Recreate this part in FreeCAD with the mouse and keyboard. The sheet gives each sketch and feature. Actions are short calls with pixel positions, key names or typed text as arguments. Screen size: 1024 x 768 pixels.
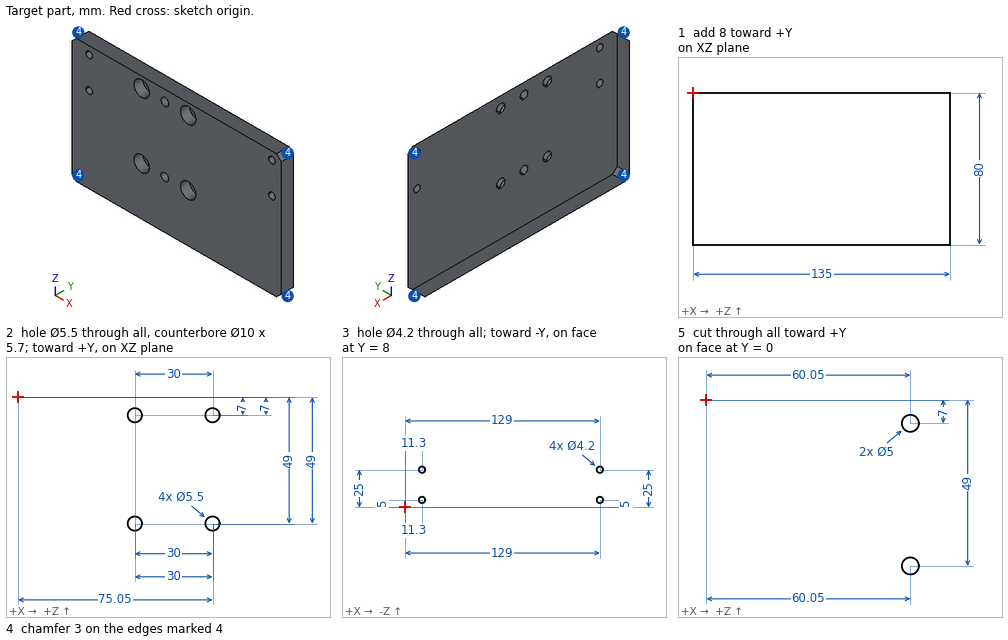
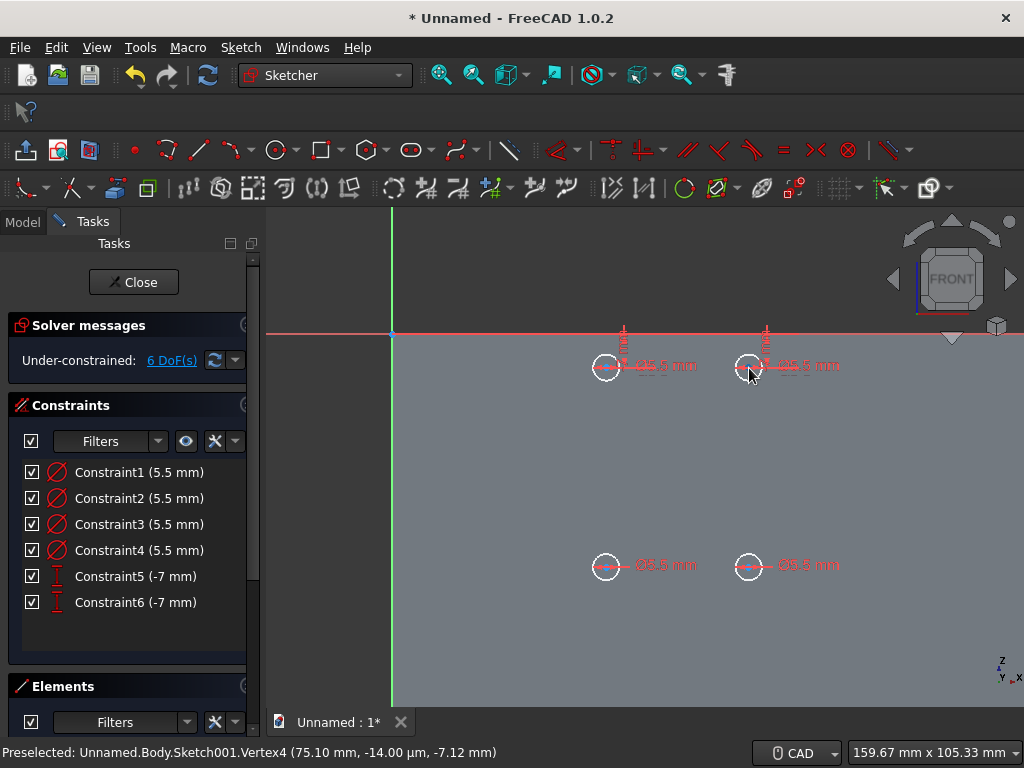
click(749, 567)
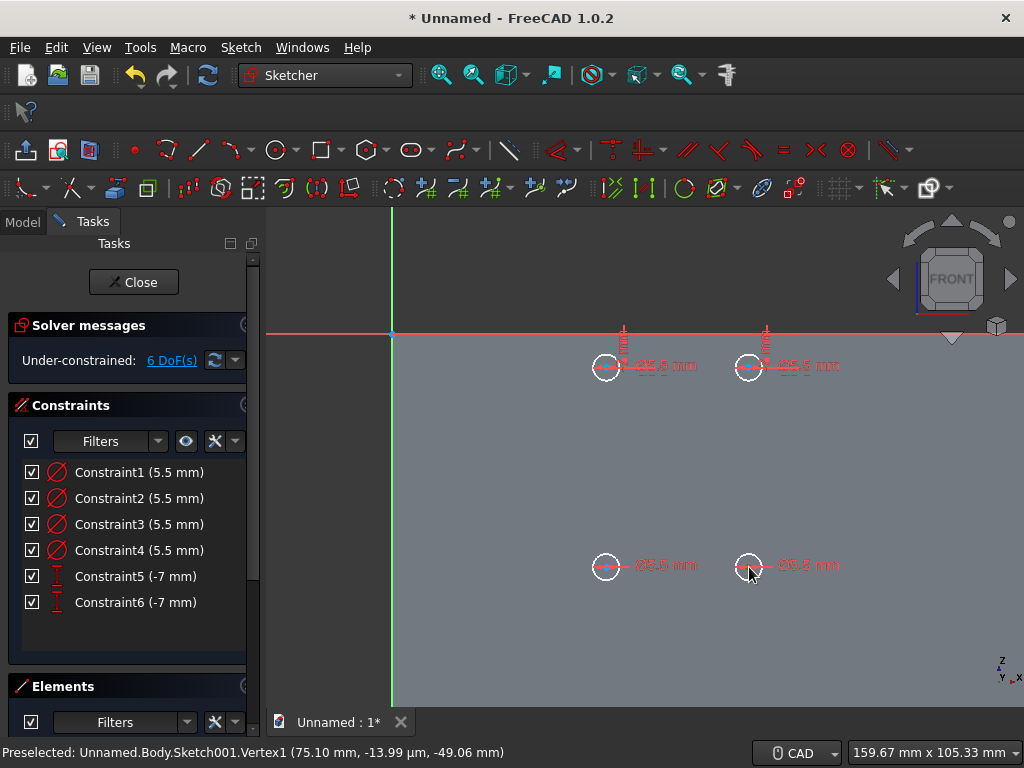
key(i)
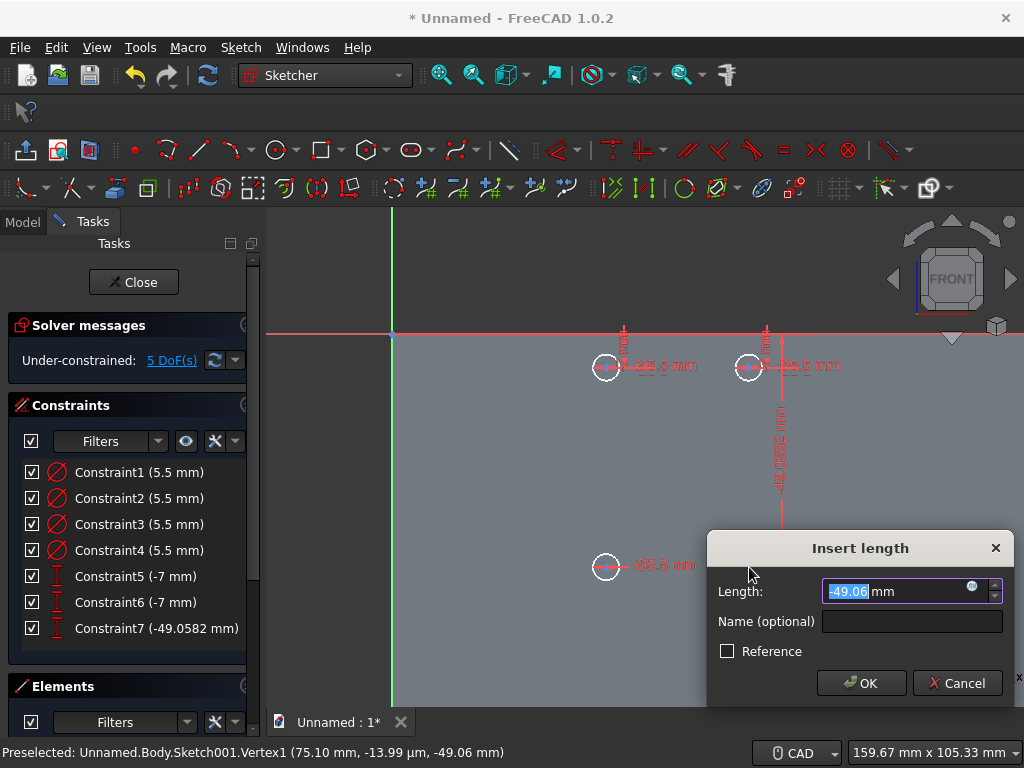
text(-49)
key(Return)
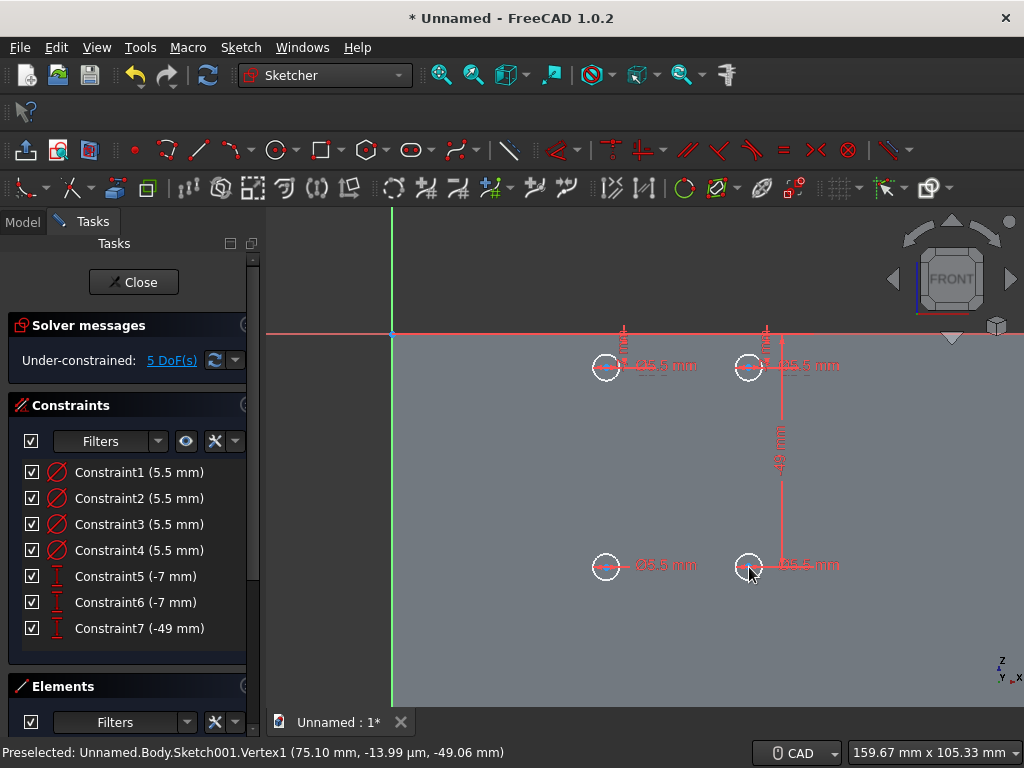
click(606, 567)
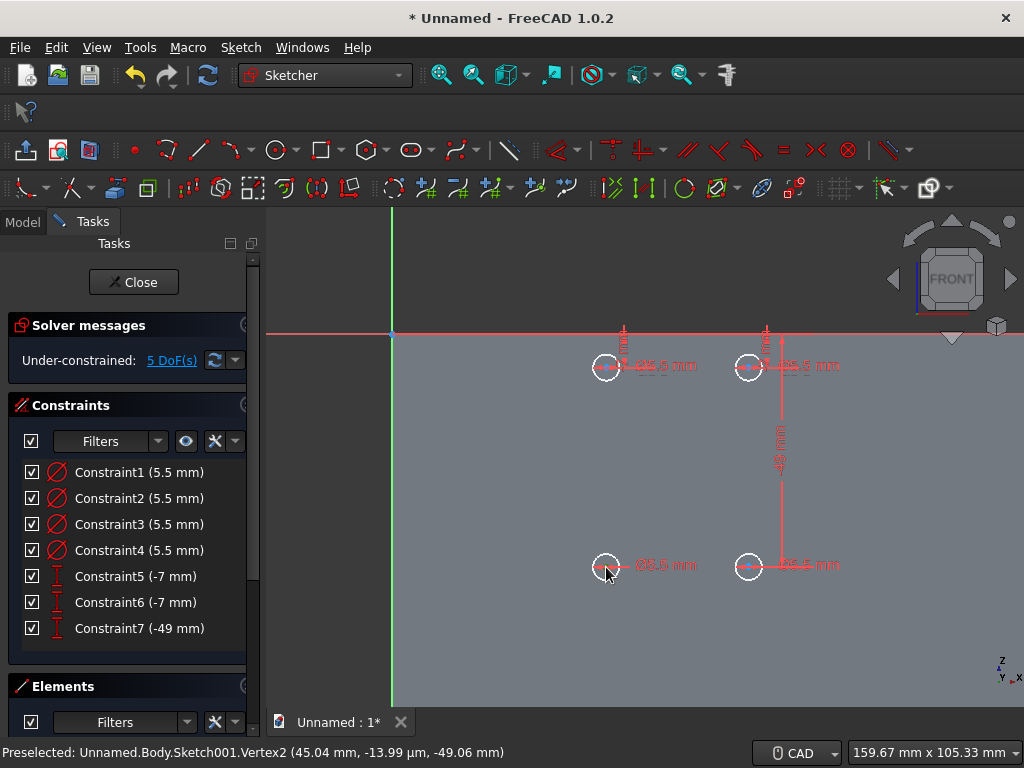
key(i)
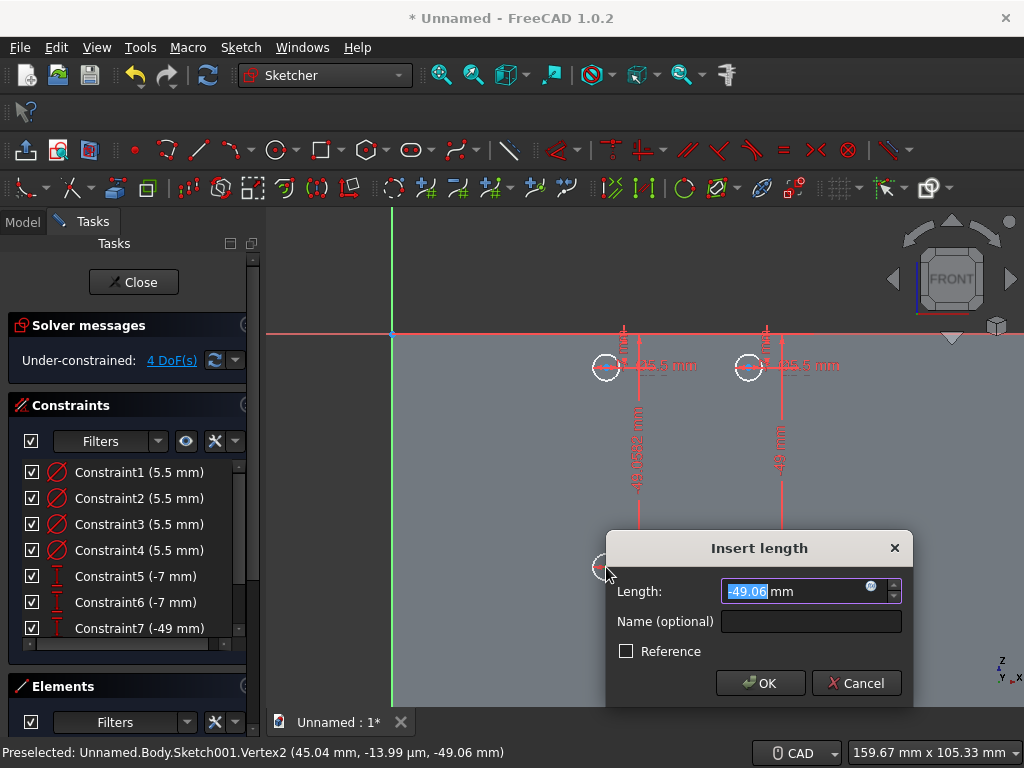
text(-49)
key(Return)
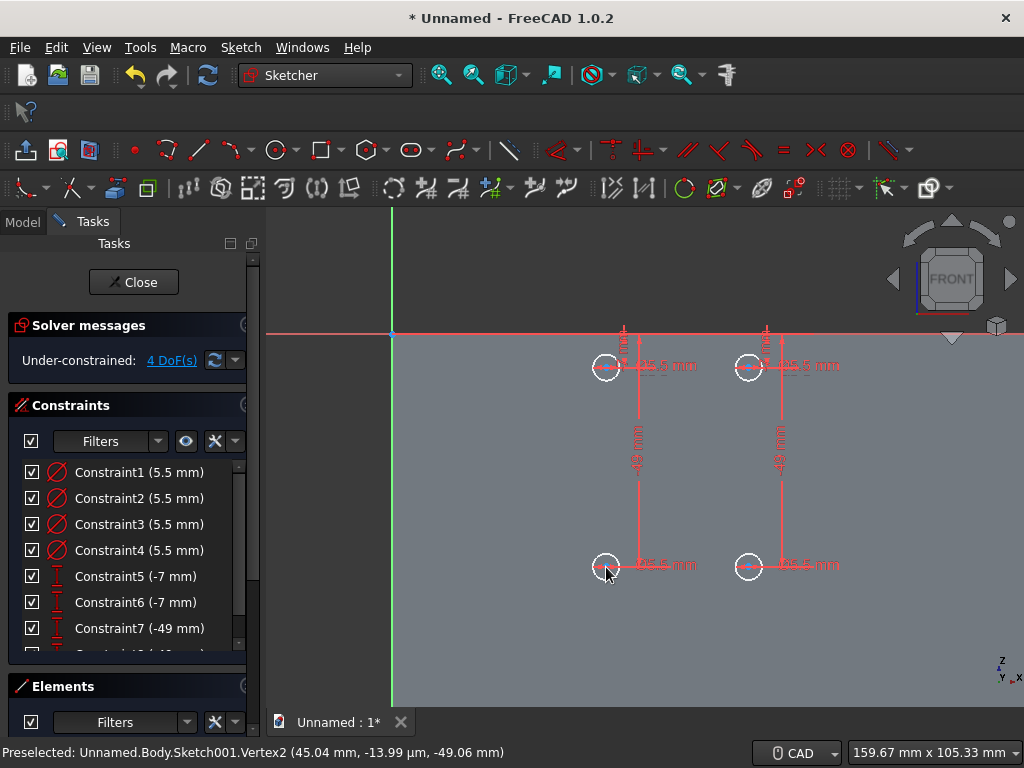
click(749, 567)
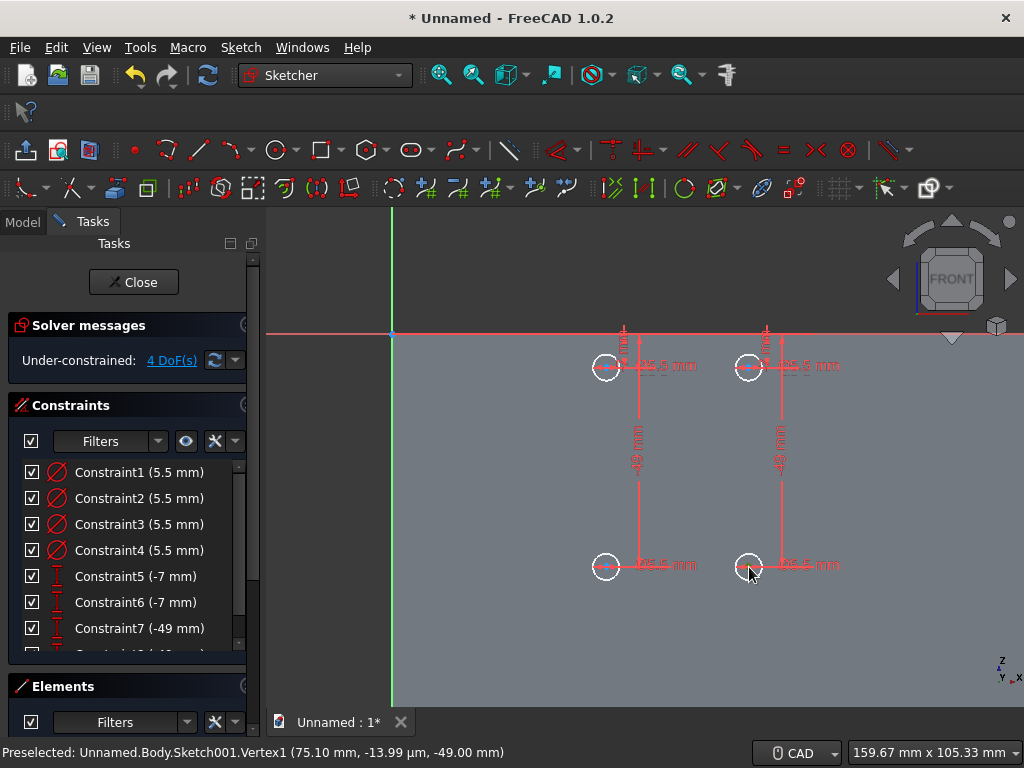
click(606, 567)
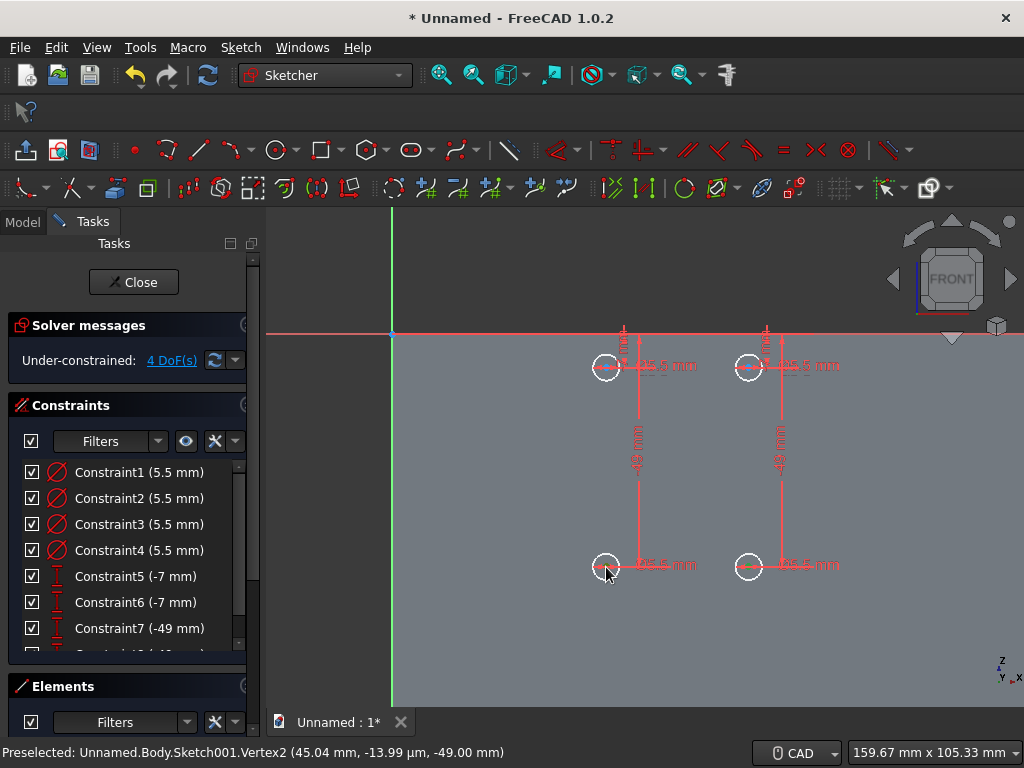
key(l)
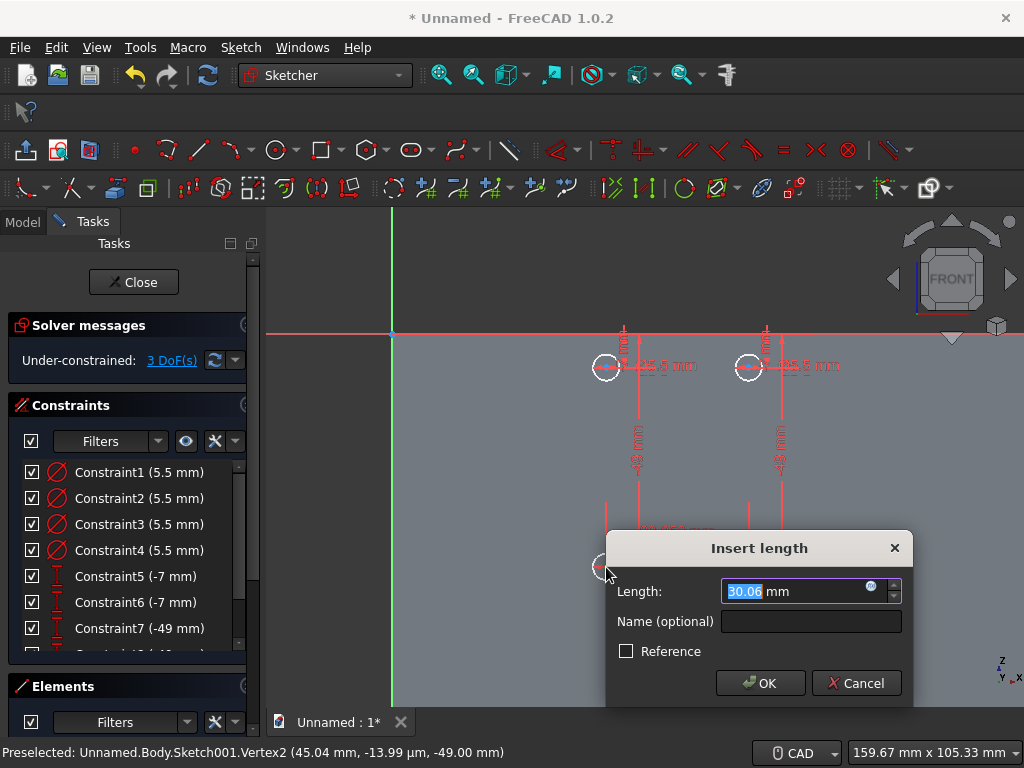
text(30)
key(Return)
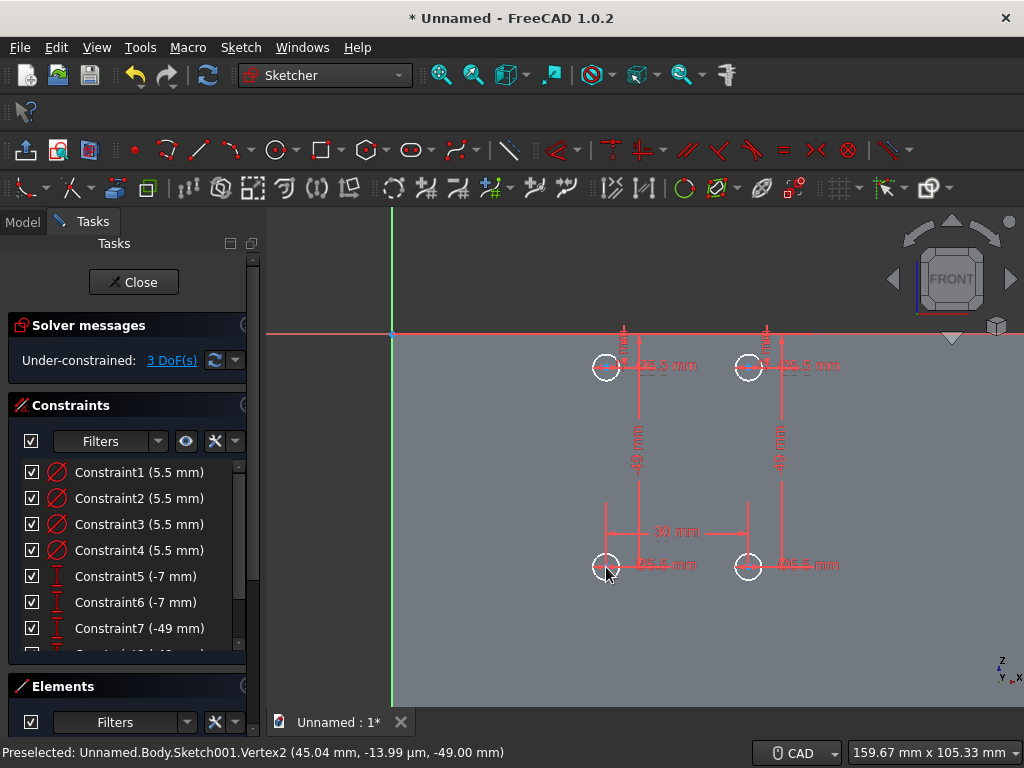
click(748, 567)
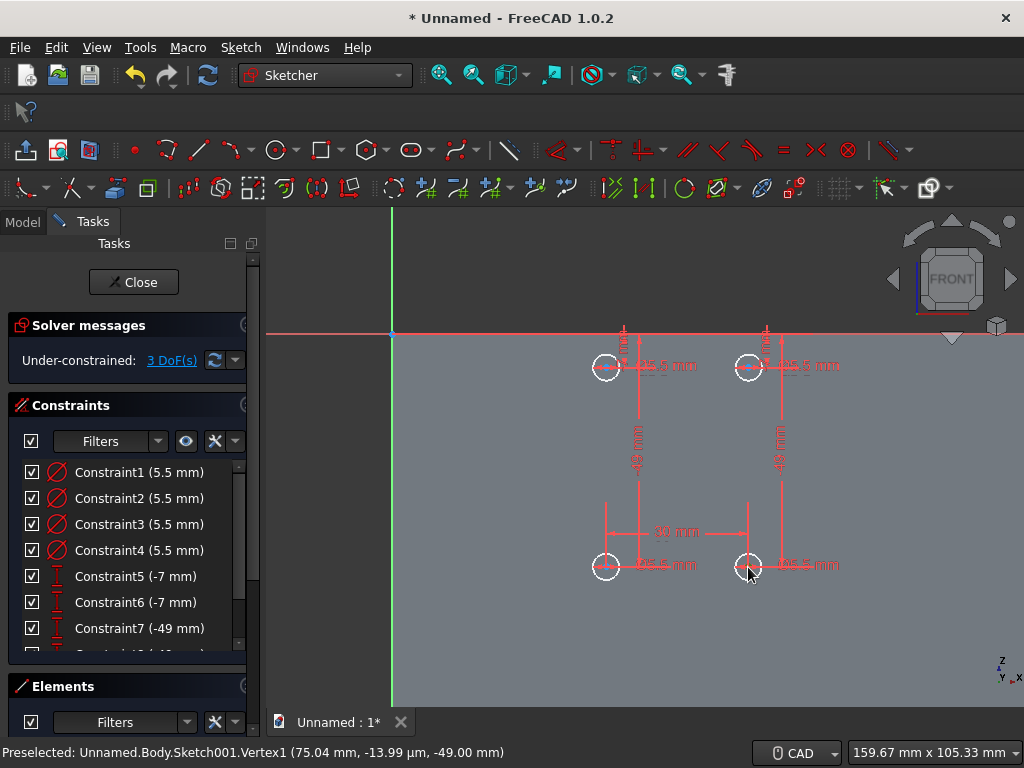
click(606, 368)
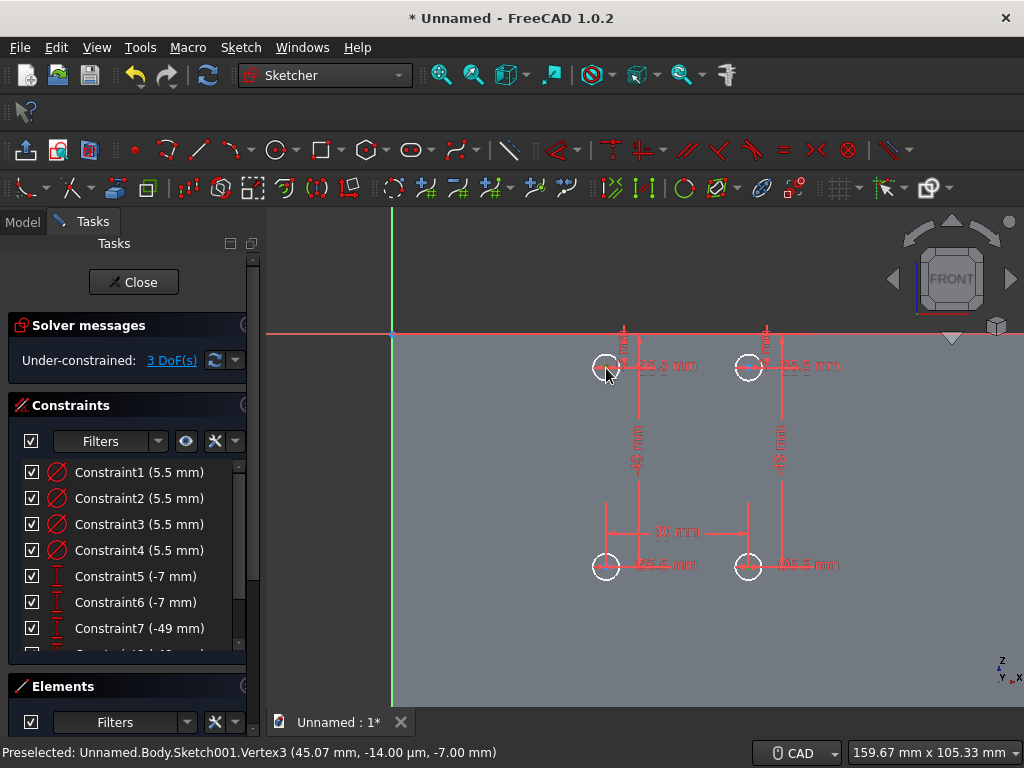
key(l)